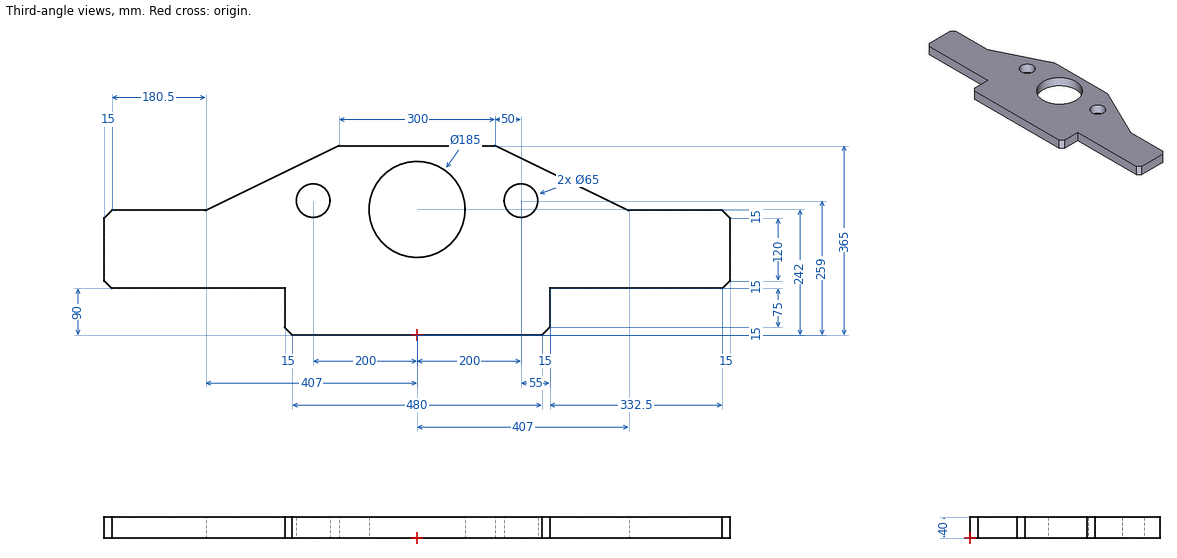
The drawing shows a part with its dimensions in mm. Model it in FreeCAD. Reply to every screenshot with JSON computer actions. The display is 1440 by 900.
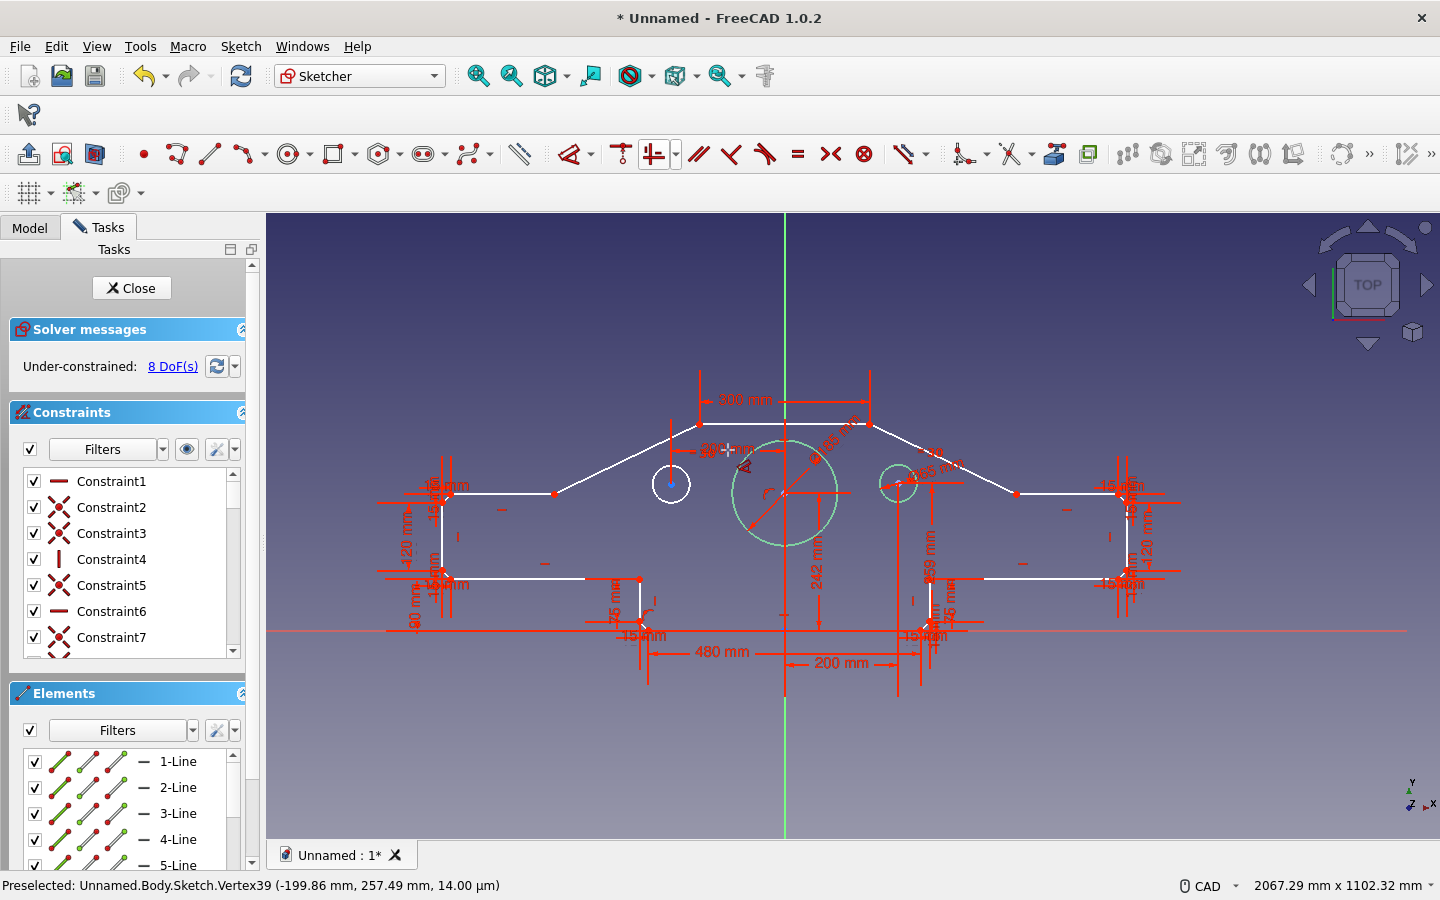
{"action": "left_click", "coordinate": [671, 484]}
{"action": "left_click", "coordinate": [637, 557]}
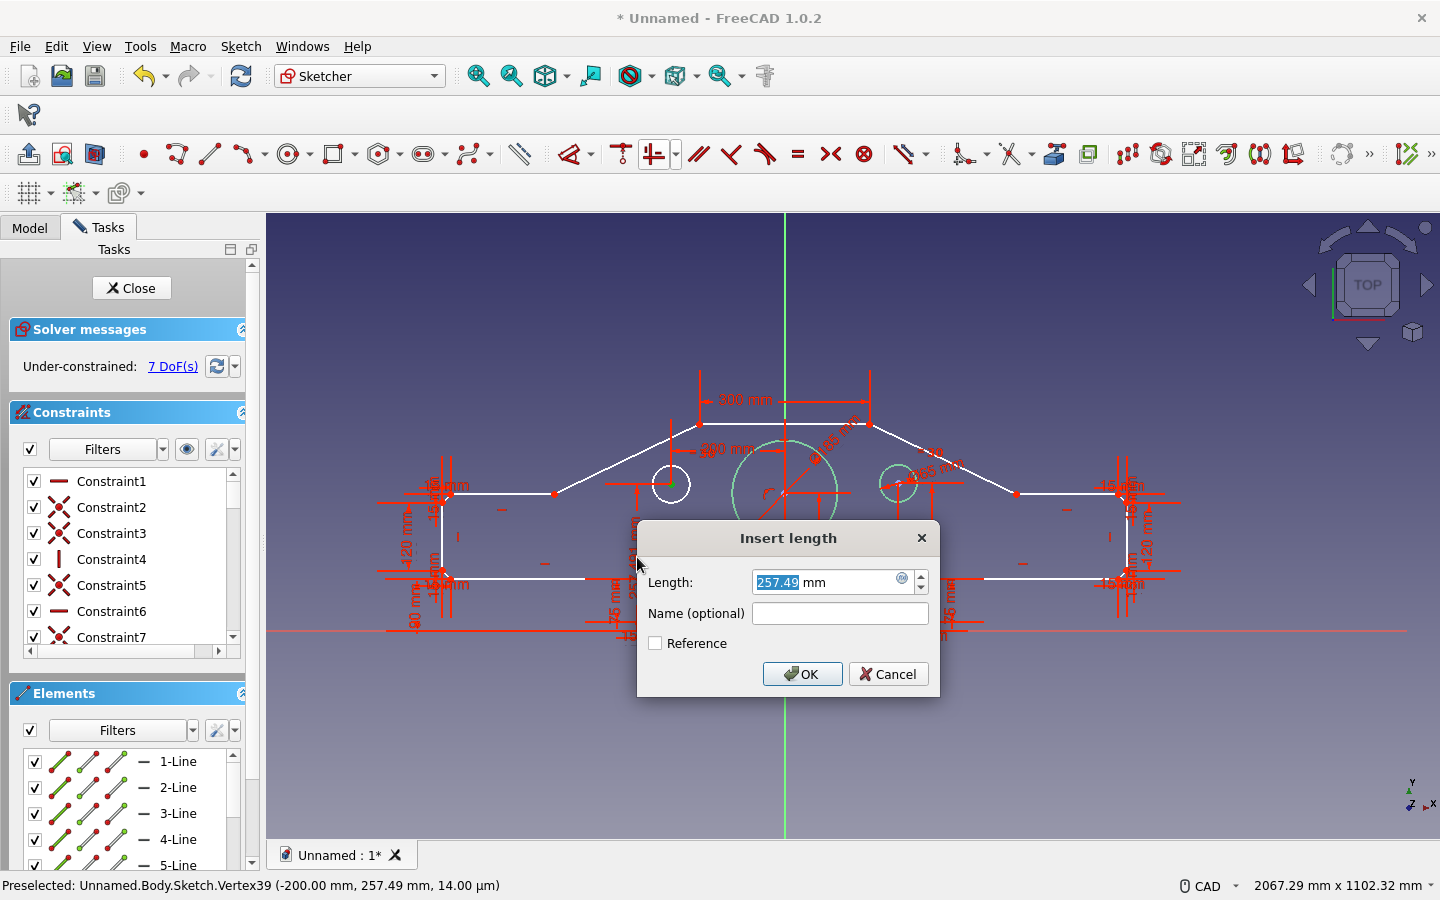
{"action": "type", "text": "259"}
{"action": "key", "text": "Return"}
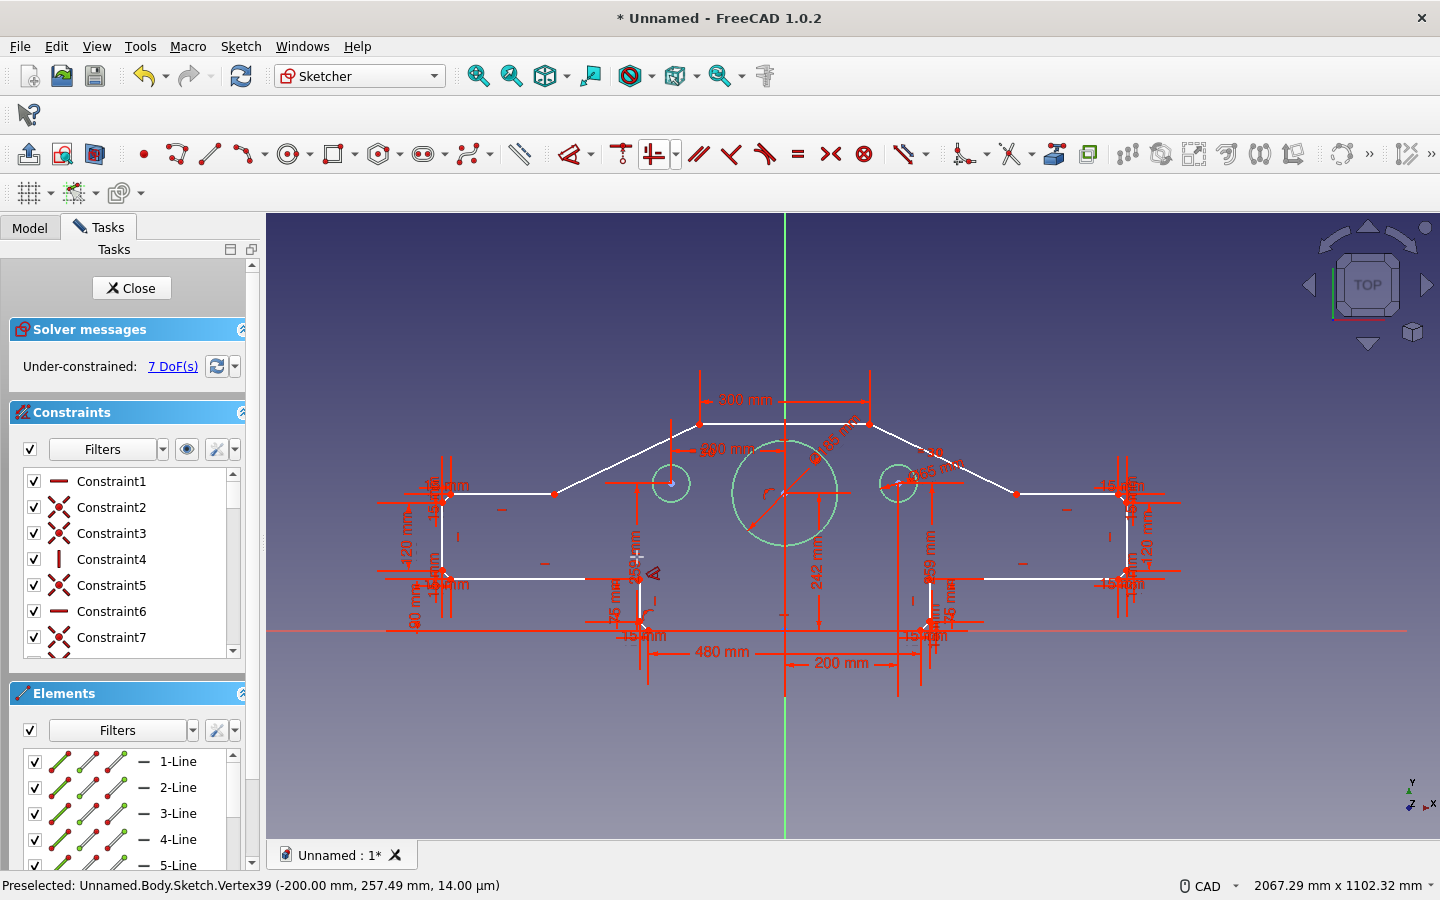
{"action": "scroll", "coordinate": [870, 424], "scroll_direction": "up", "scroll_amount": 2}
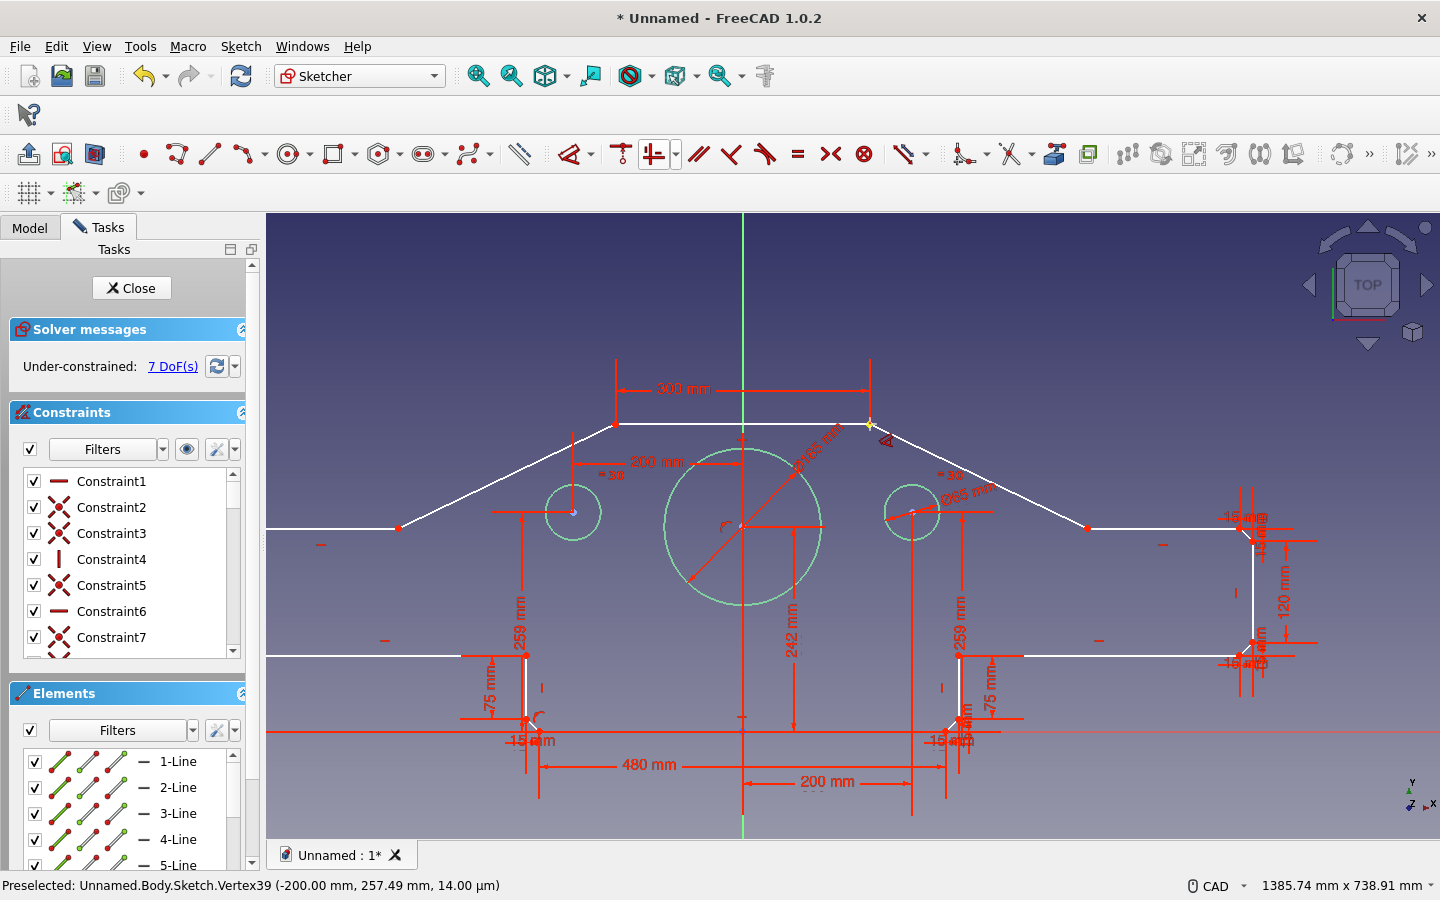
{"action": "left_click", "coordinate": [870, 424]}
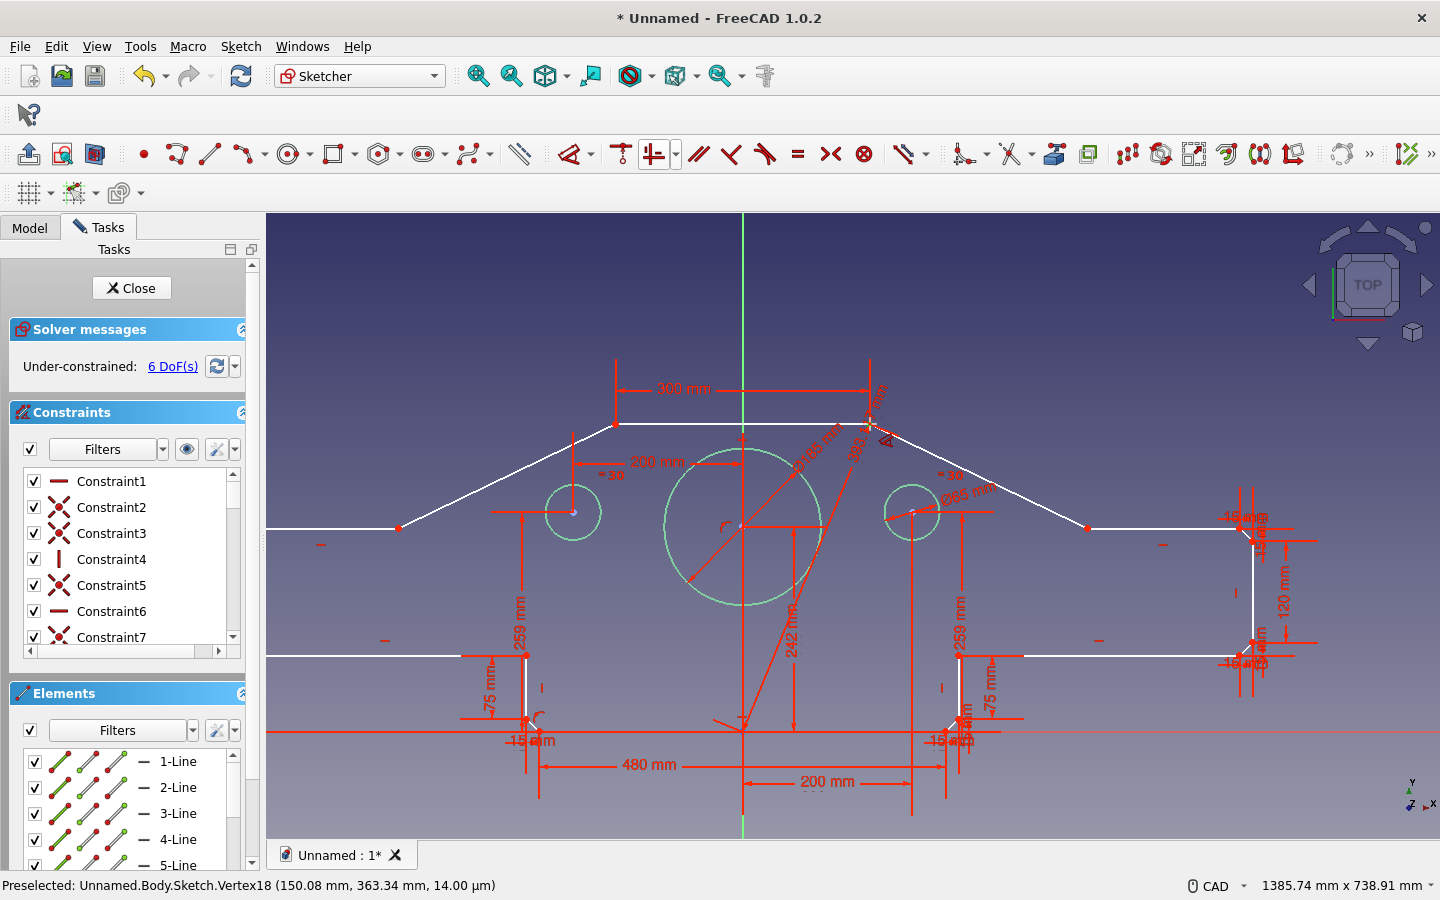
{"action": "left_click", "coordinate": [912, 512]}
{"action": "left_click", "coordinate": [891, 390]}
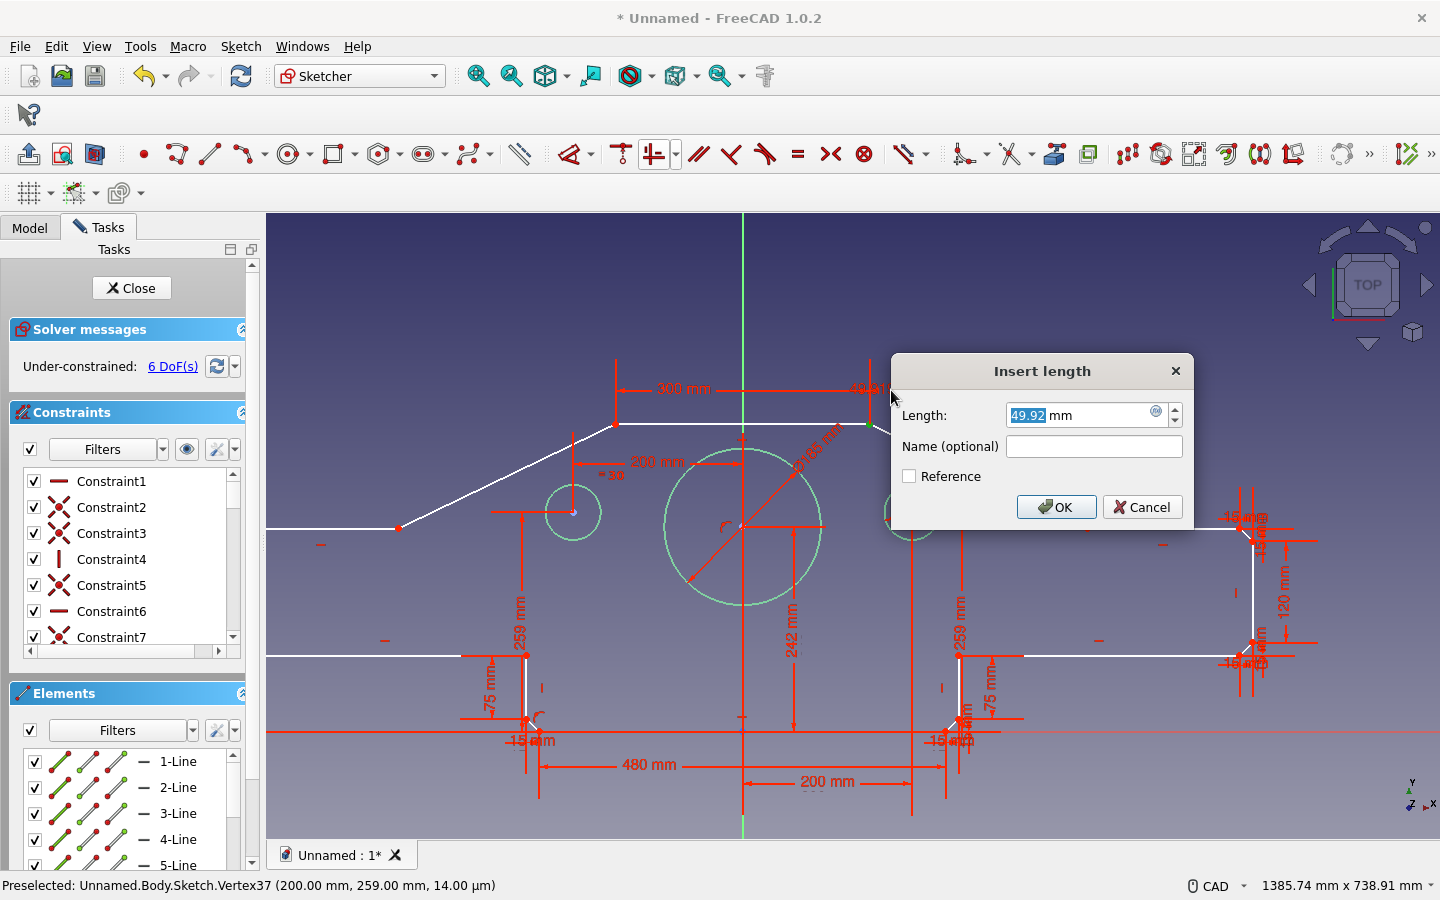
{"action": "type", "text": "50"}
{"action": "key", "text": "Return"}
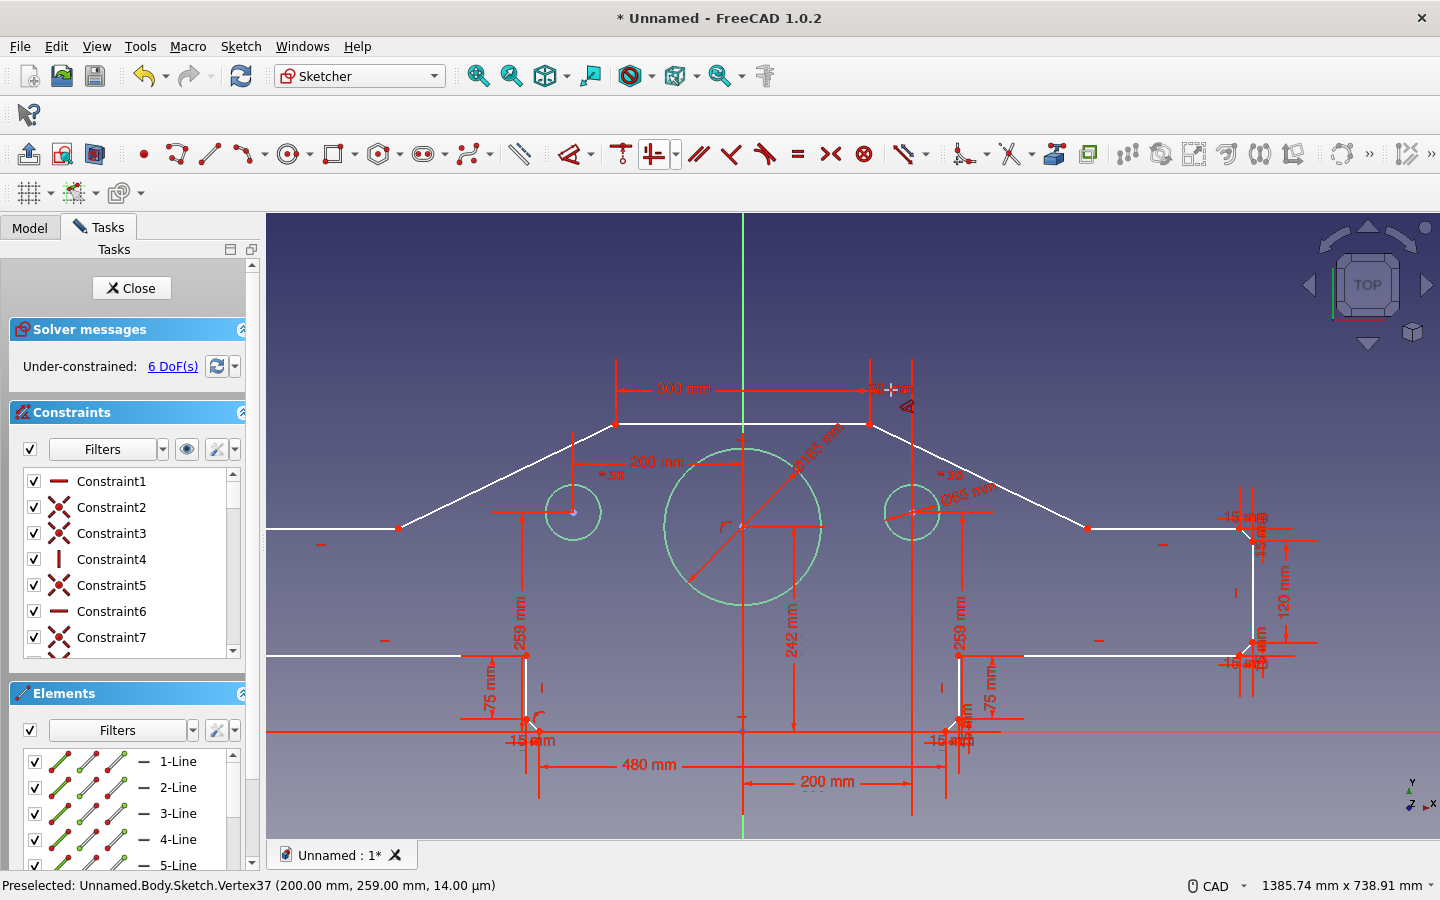
{"action": "left_click", "coordinate": [959, 656]}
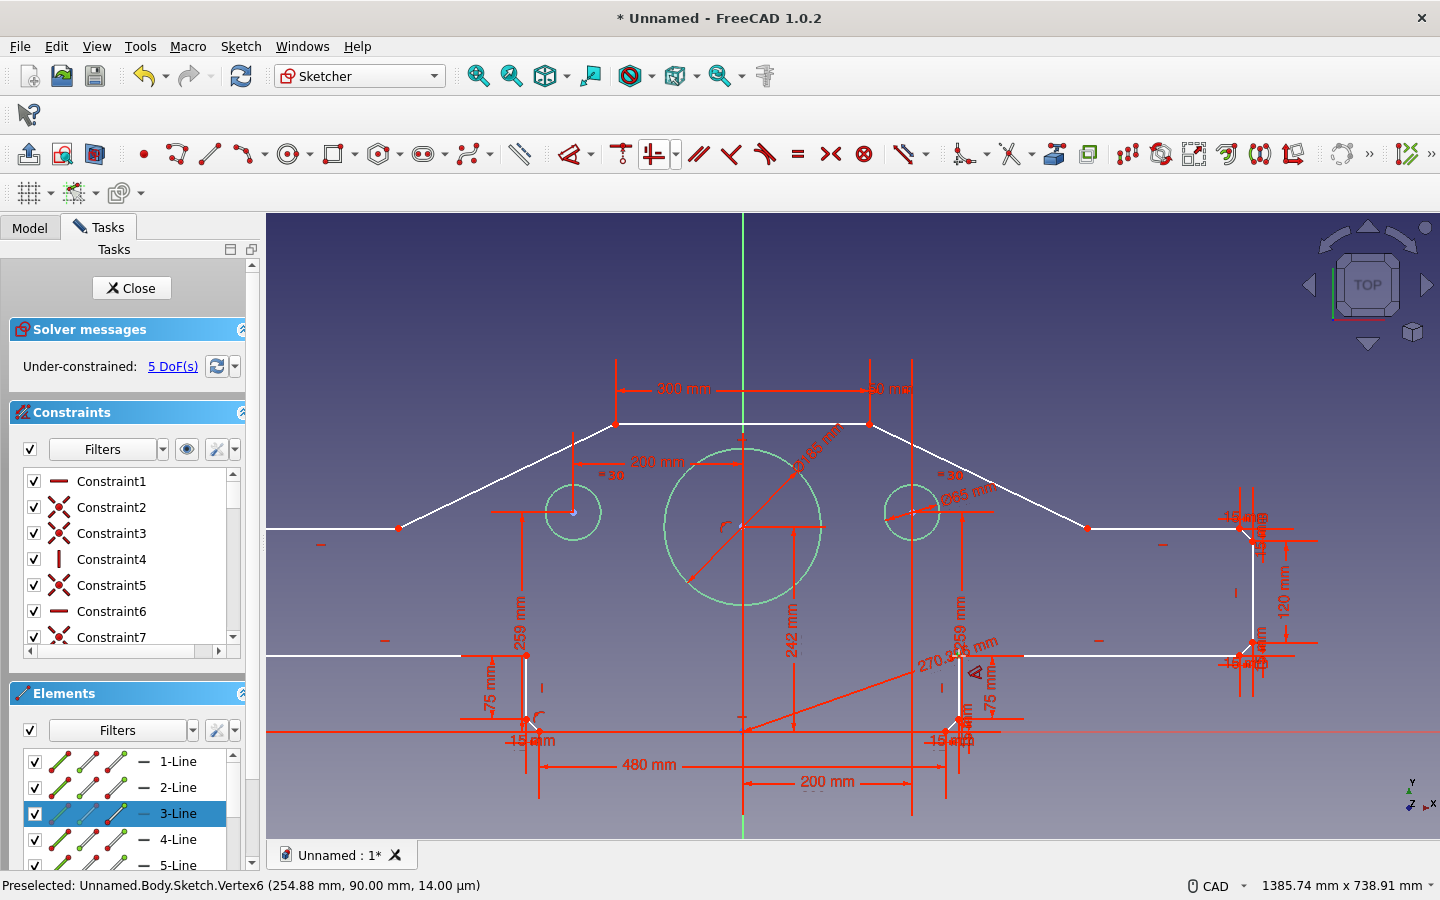
{"action": "left_click", "coordinate": [912, 512]}
{"action": "left_click", "coordinate": [919, 690]}